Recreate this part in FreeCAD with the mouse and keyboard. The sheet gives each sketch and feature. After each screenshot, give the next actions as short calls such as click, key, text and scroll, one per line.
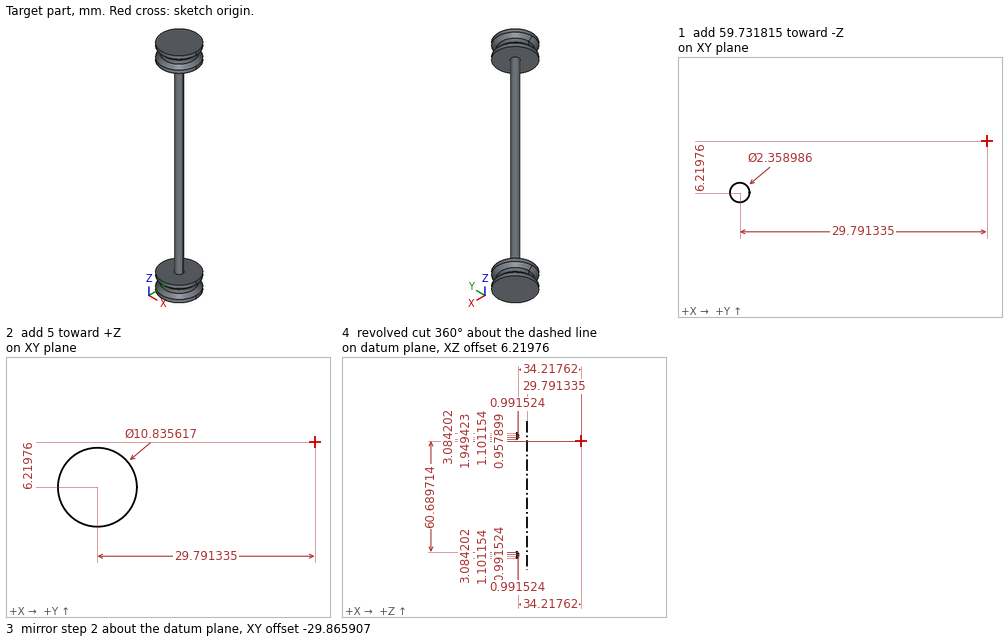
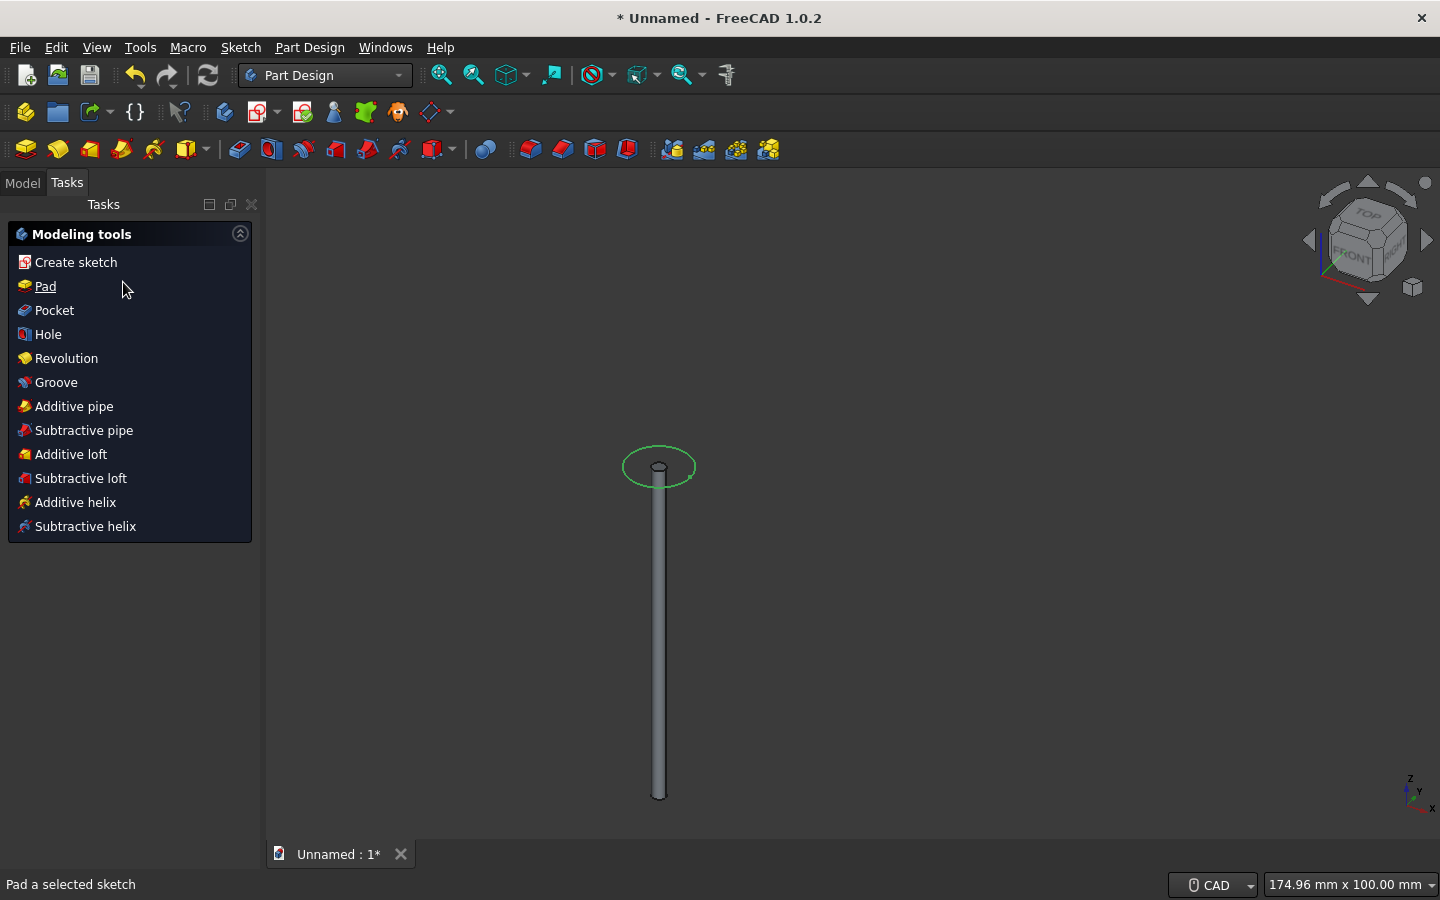
click(26, 150)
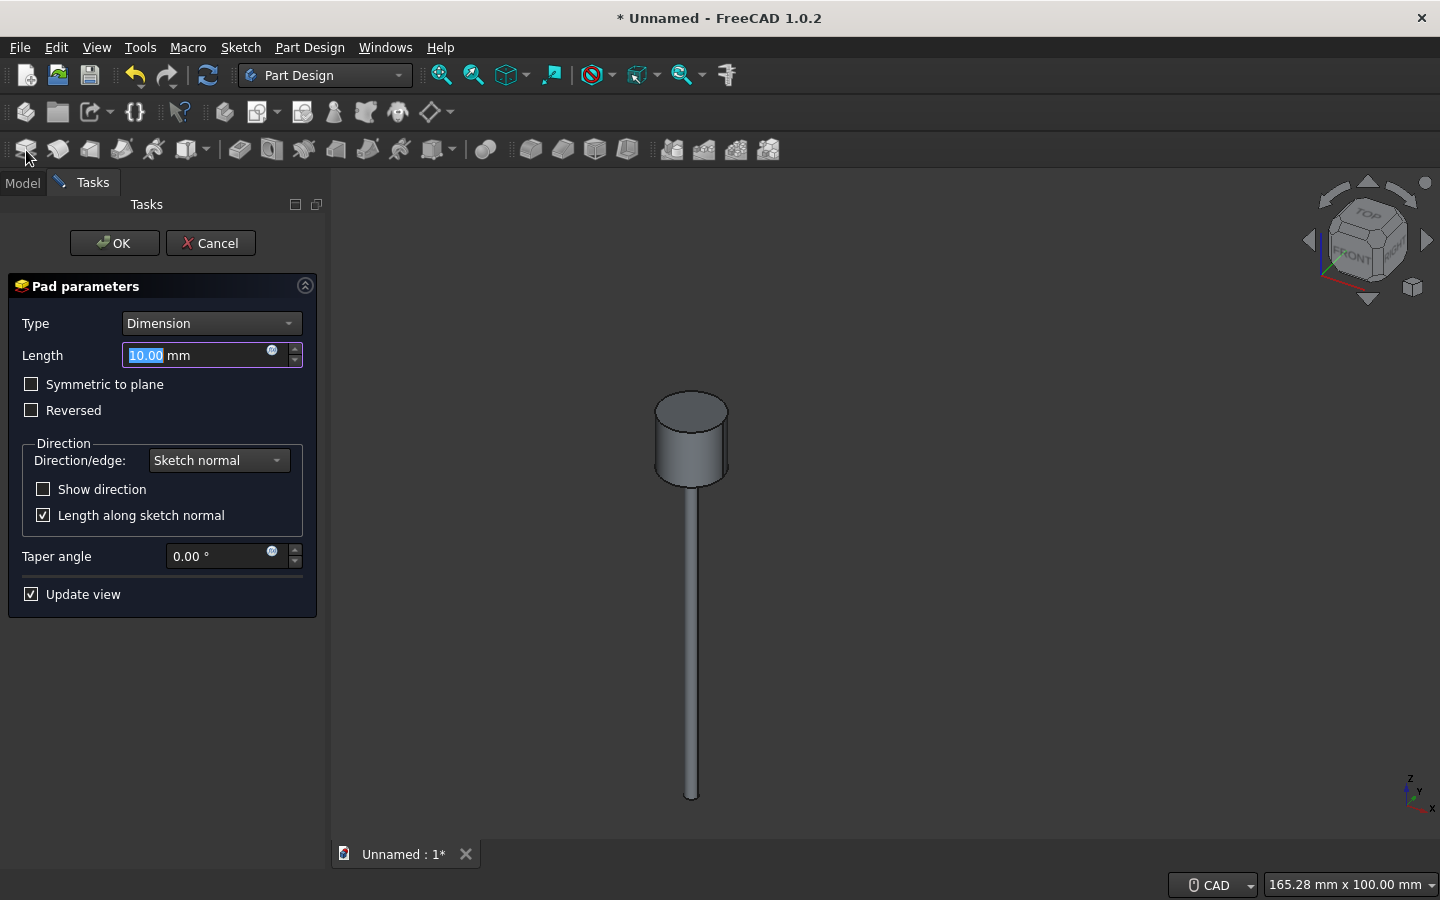
text(5)
key(Tab)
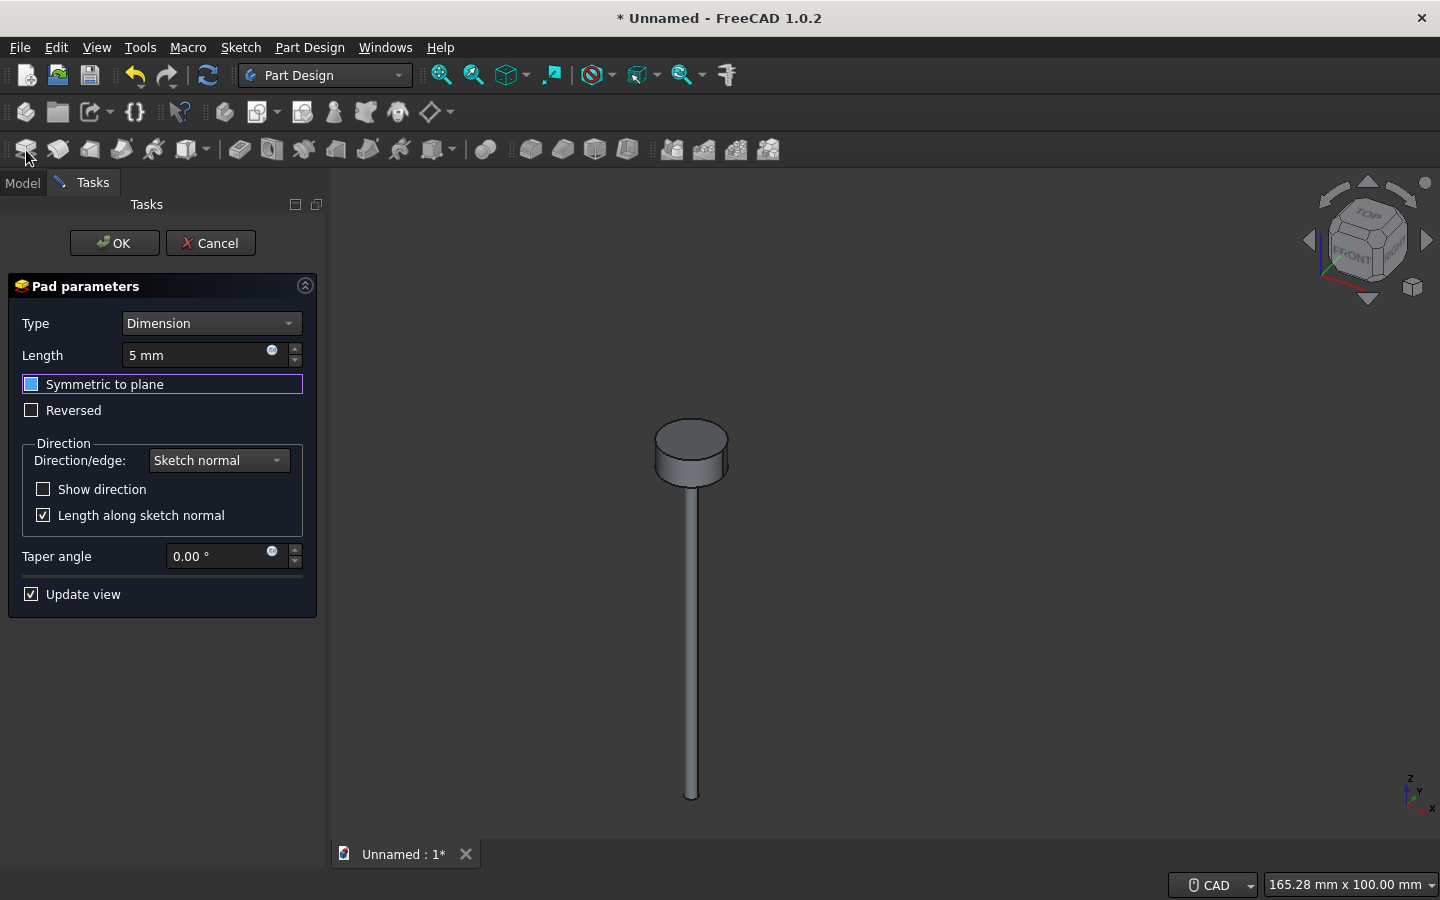
click(115, 243)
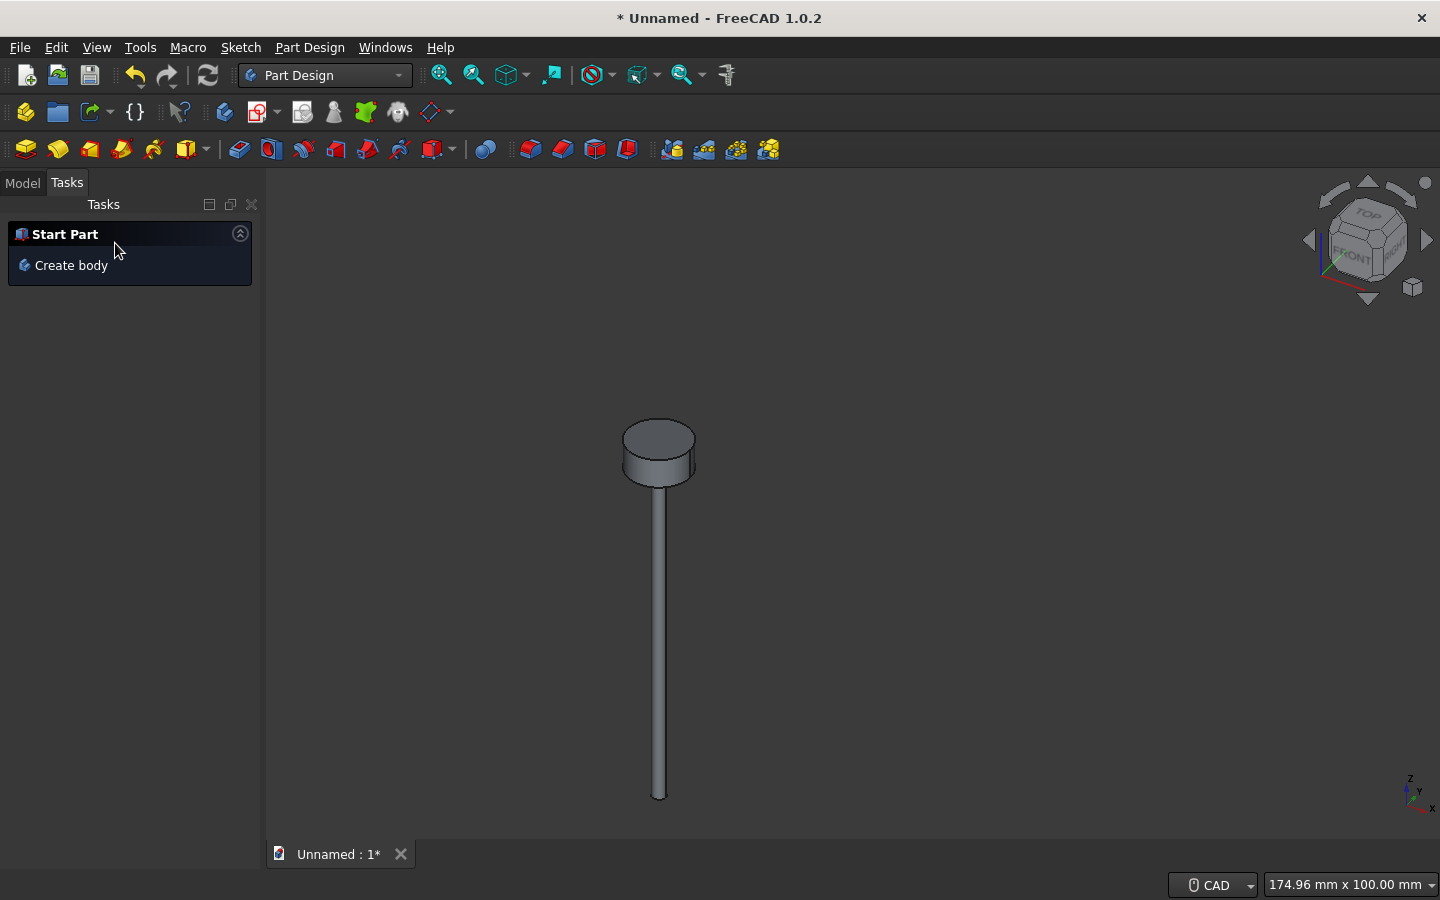
click(23, 182)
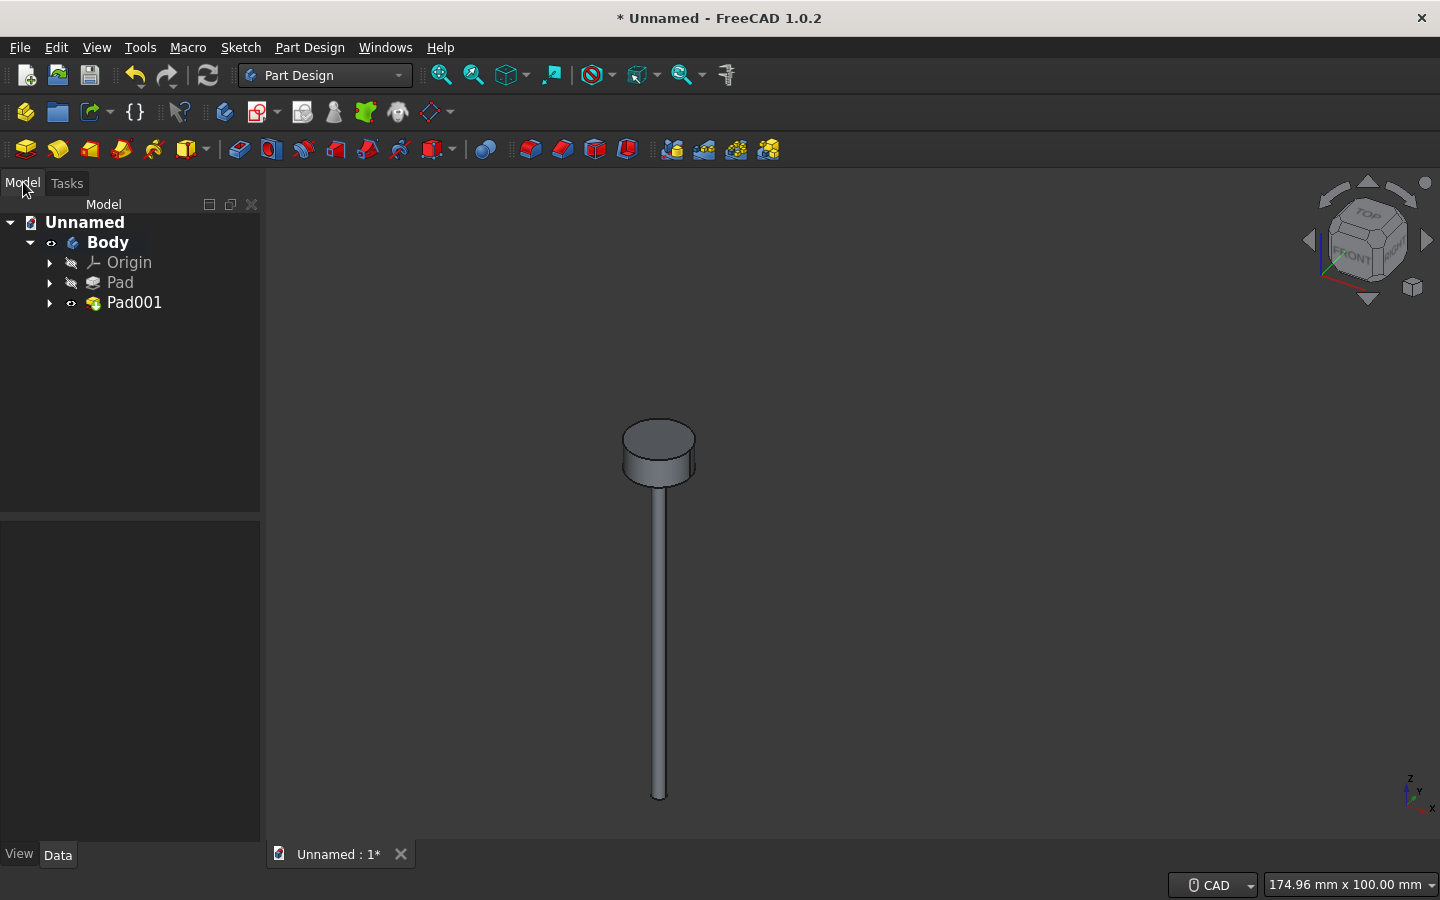
click(50, 263)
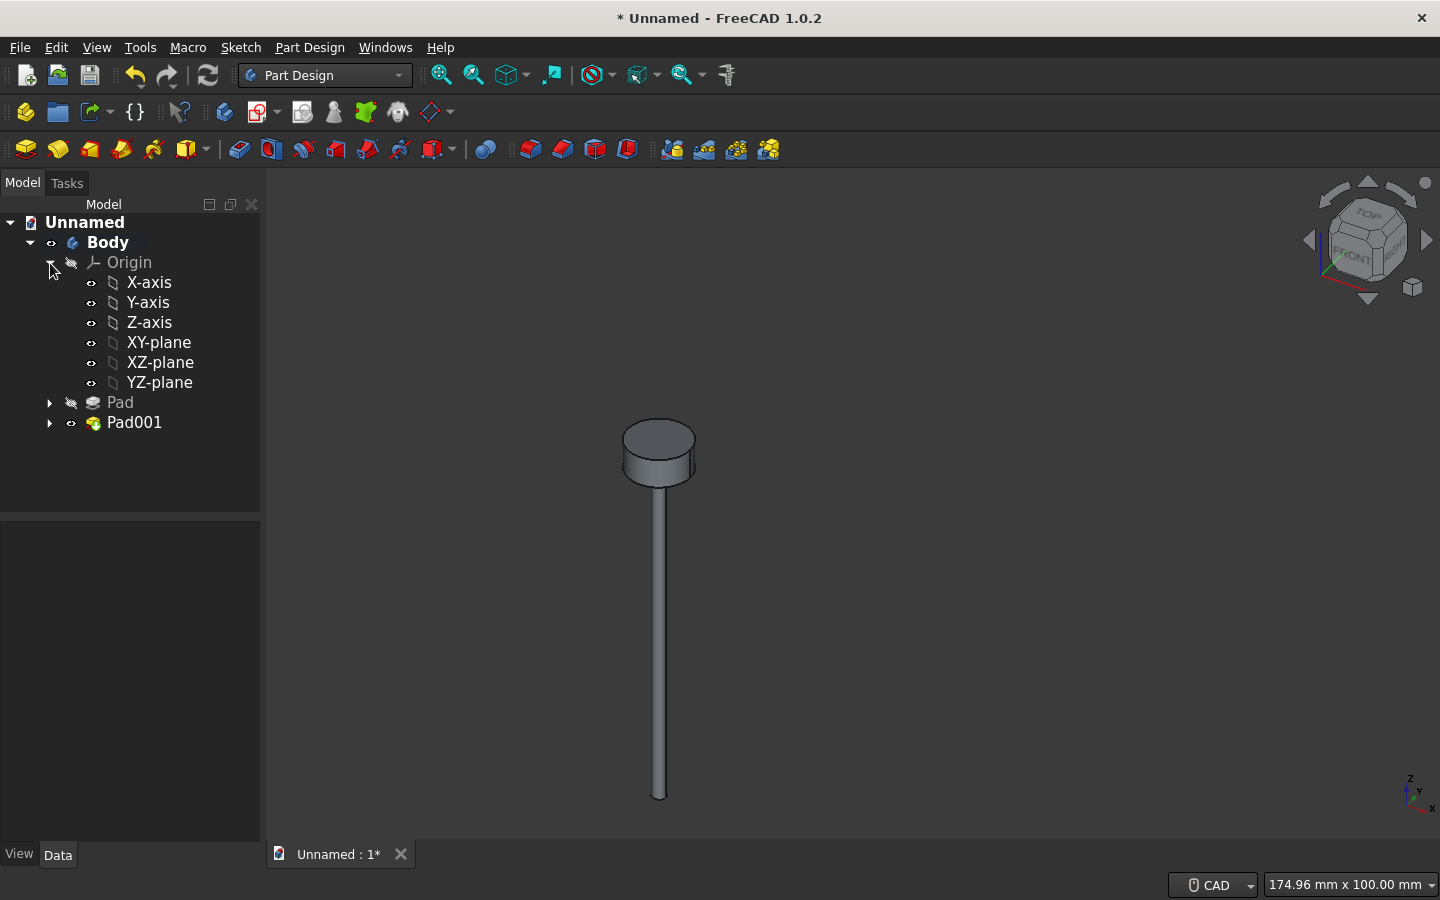
click(136, 343)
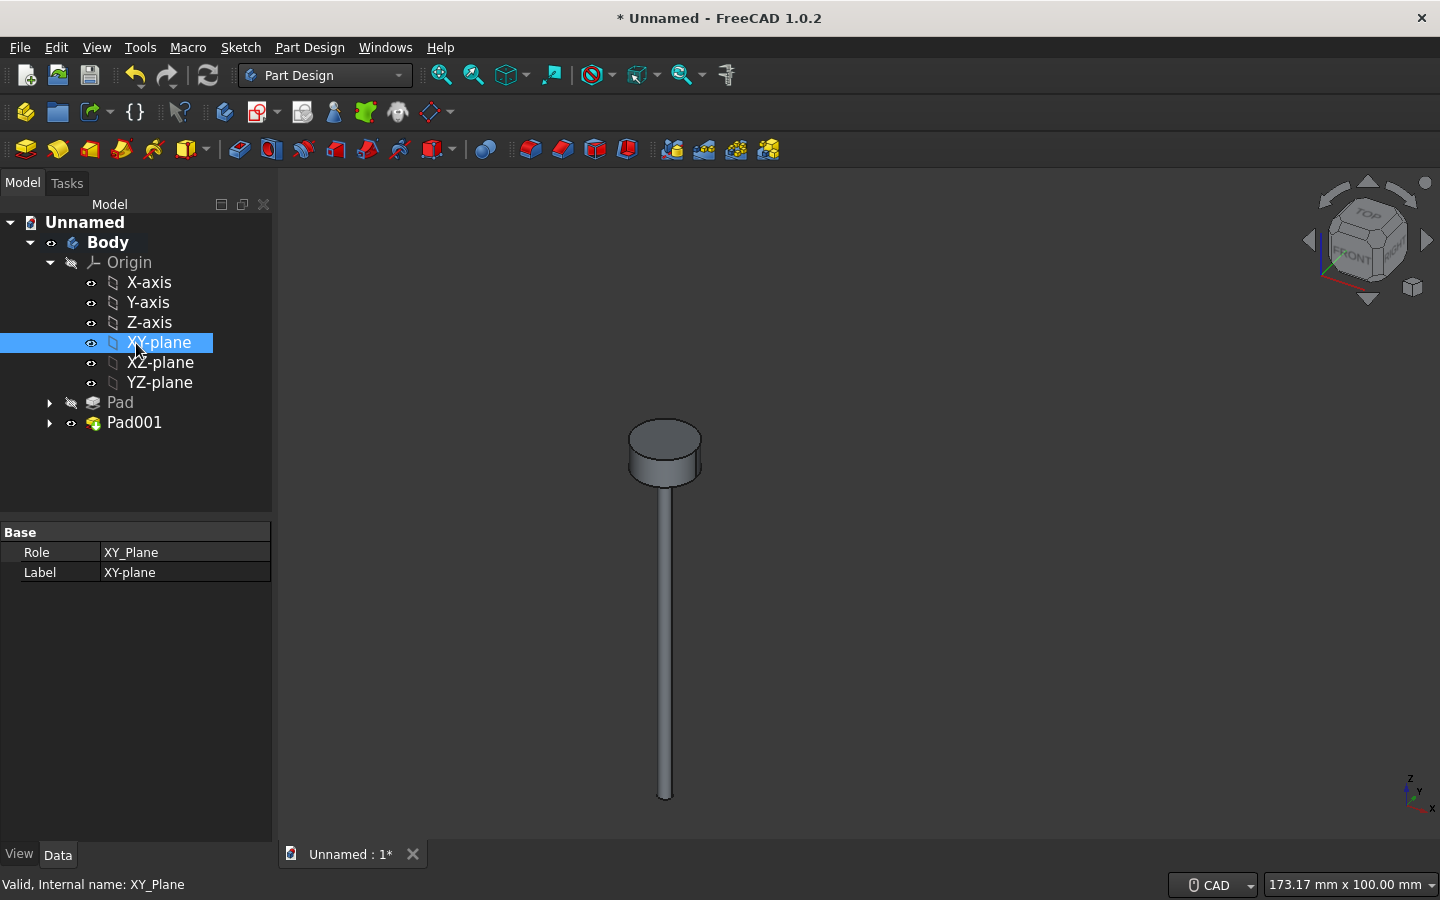
click(430, 112)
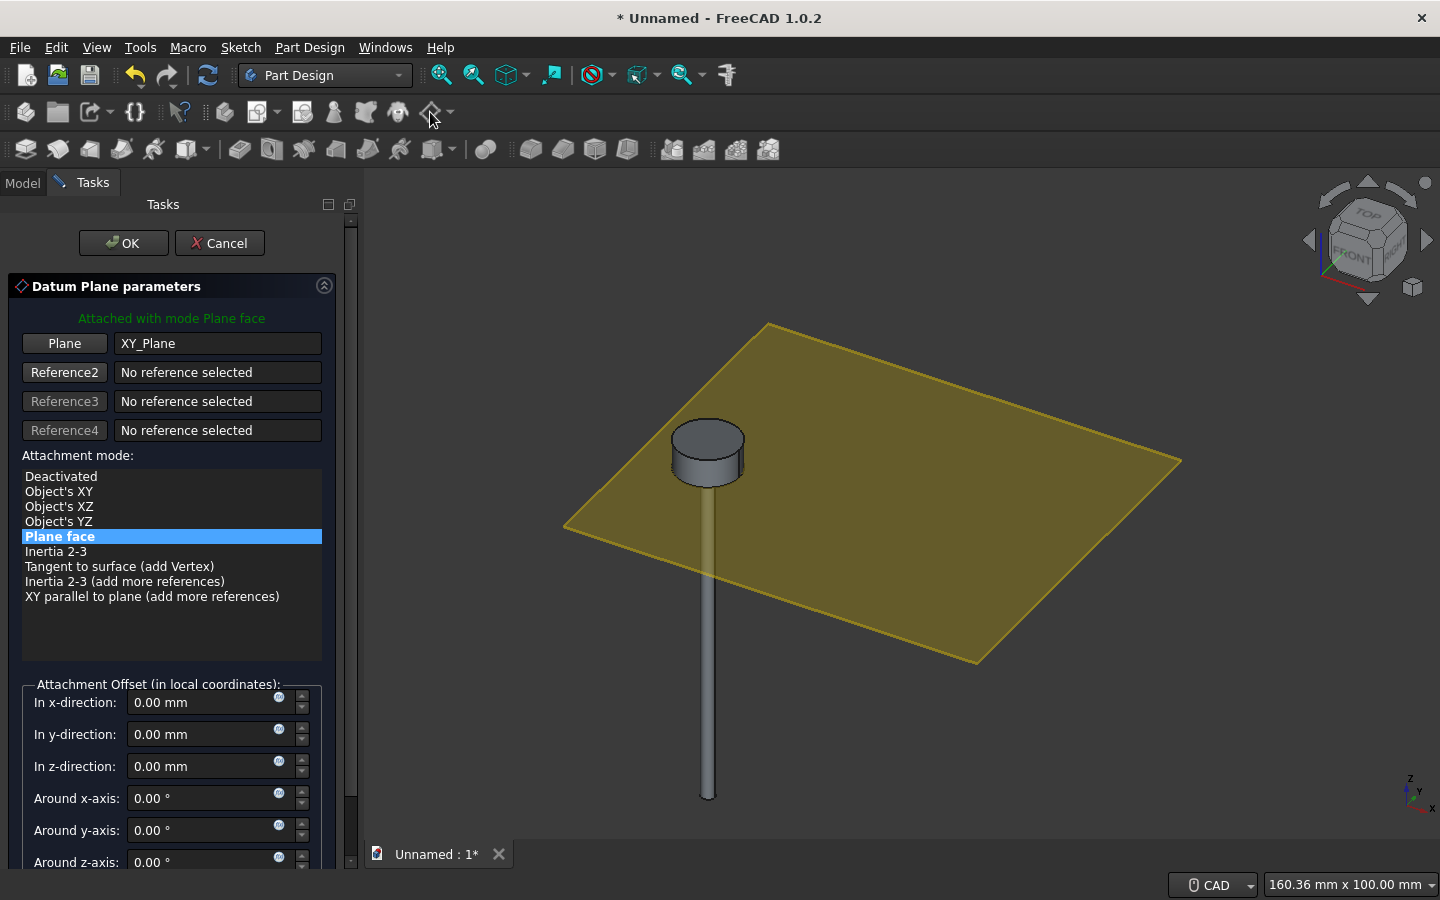
triple_click(210, 766)